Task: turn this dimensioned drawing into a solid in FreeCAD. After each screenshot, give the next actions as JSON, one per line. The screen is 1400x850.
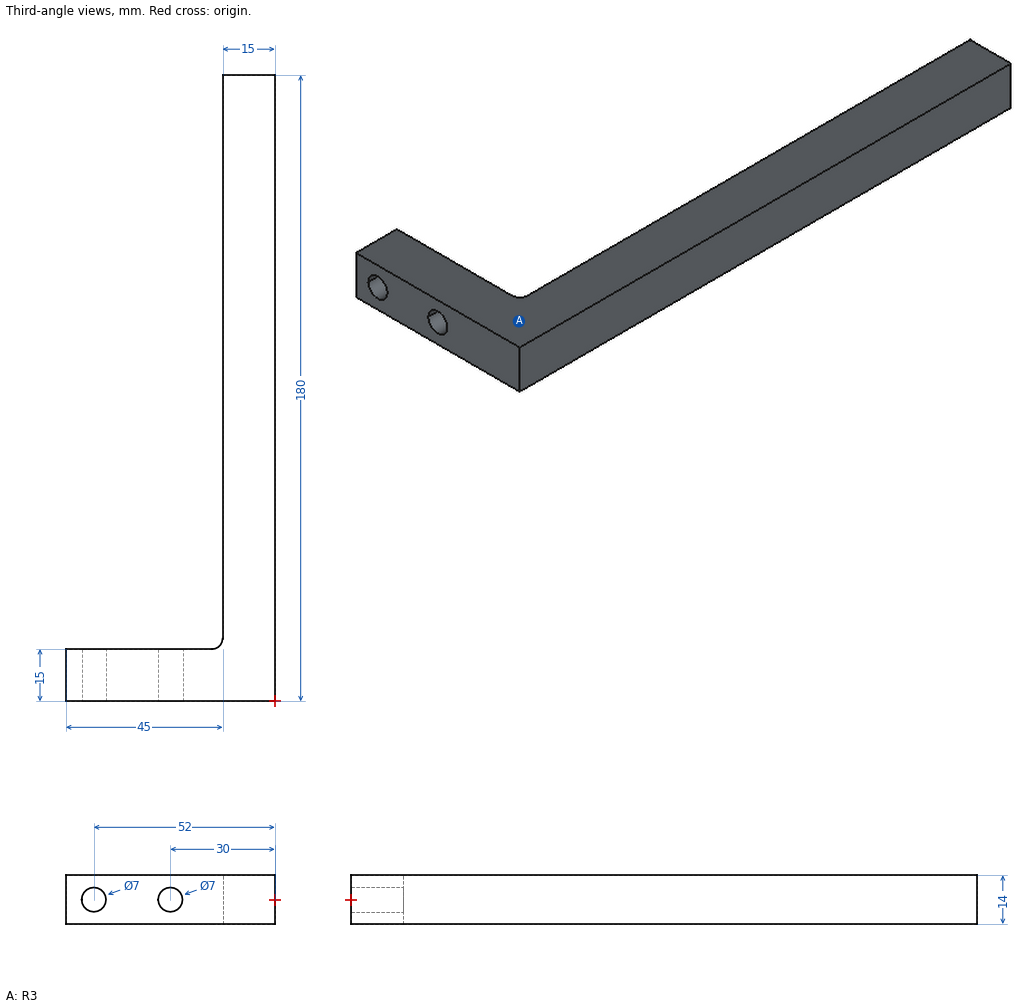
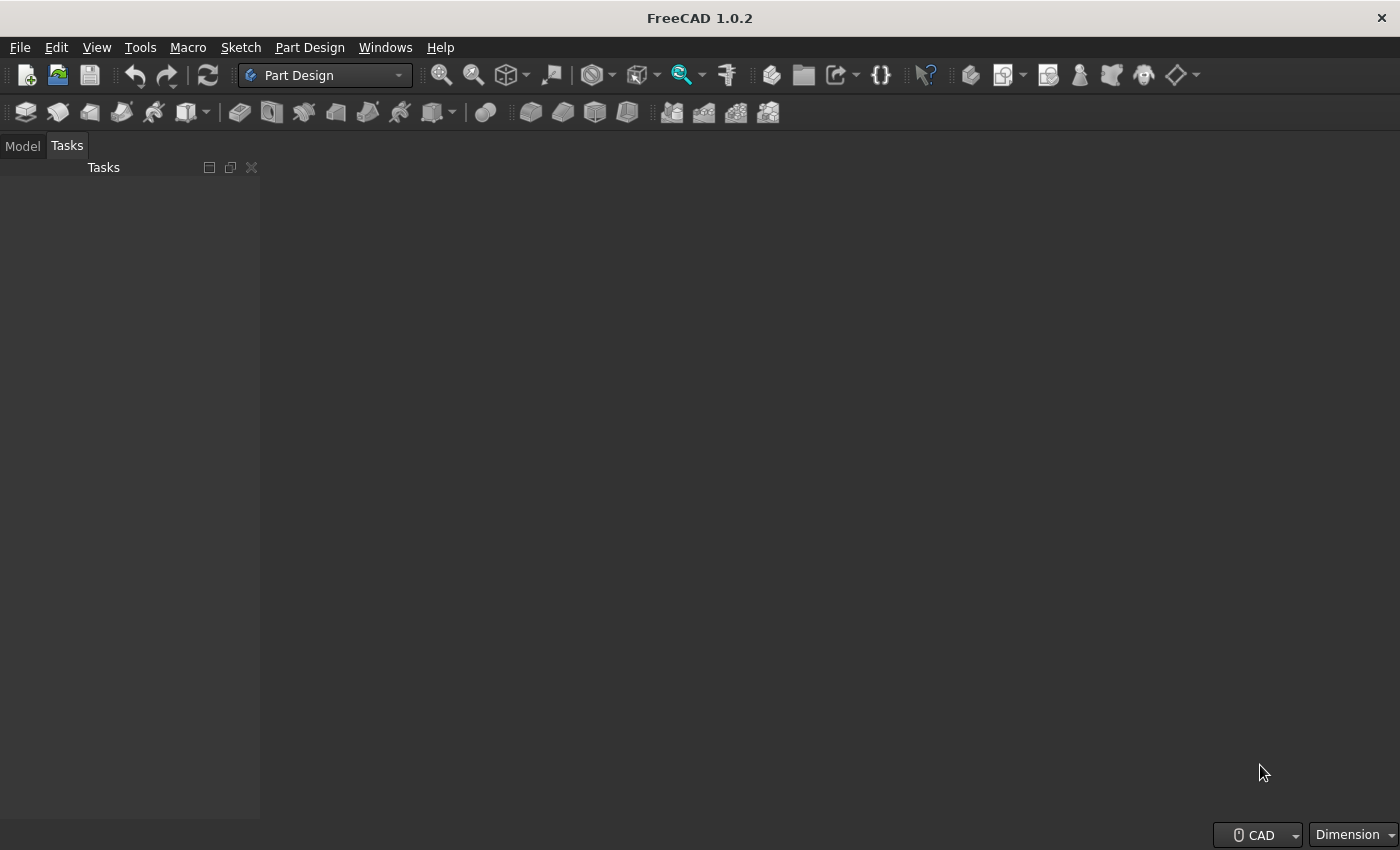
{"action": "left_click", "coordinate": [26, 76]}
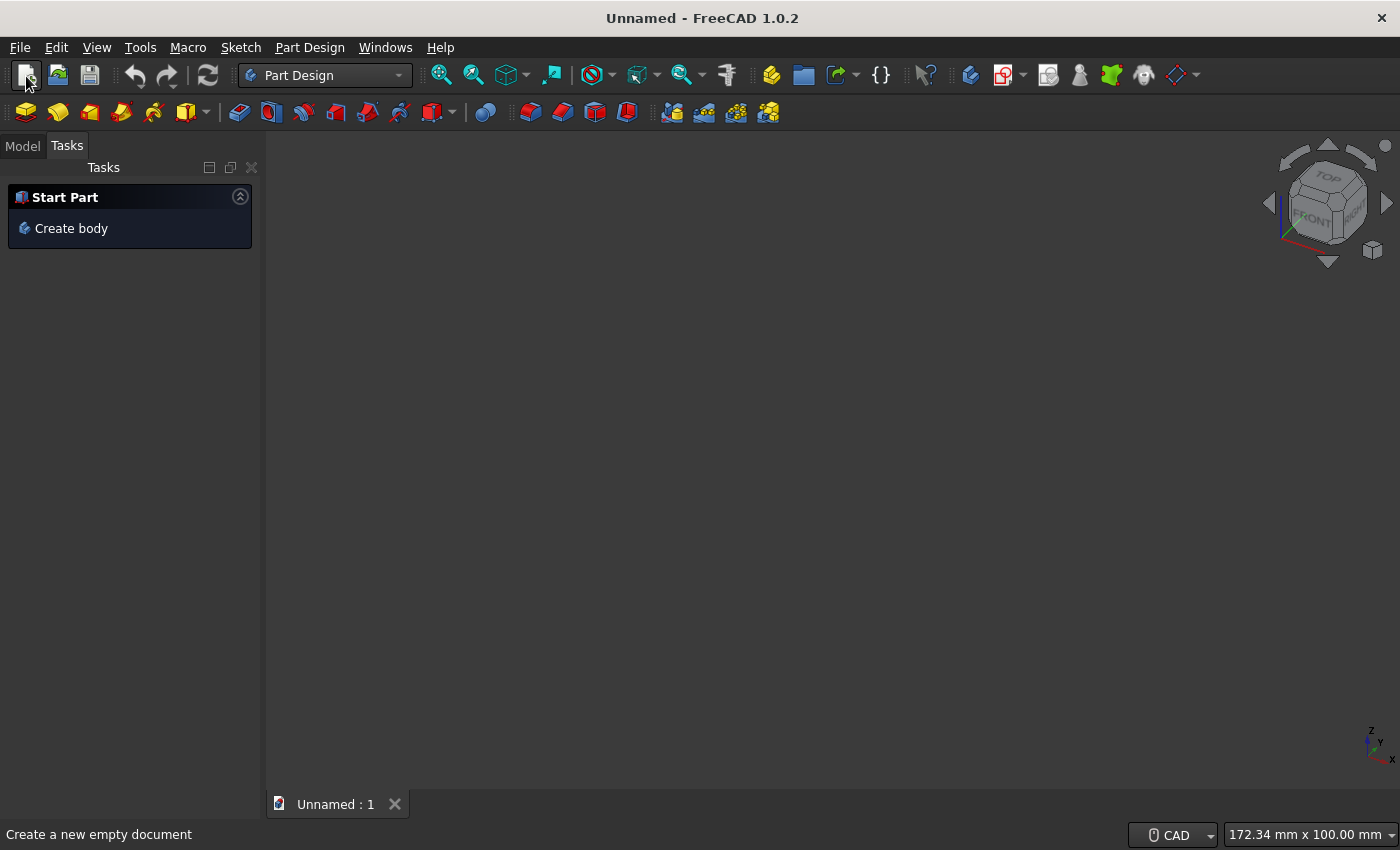
{"action": "left_click", "coordinate": [1004, 76]}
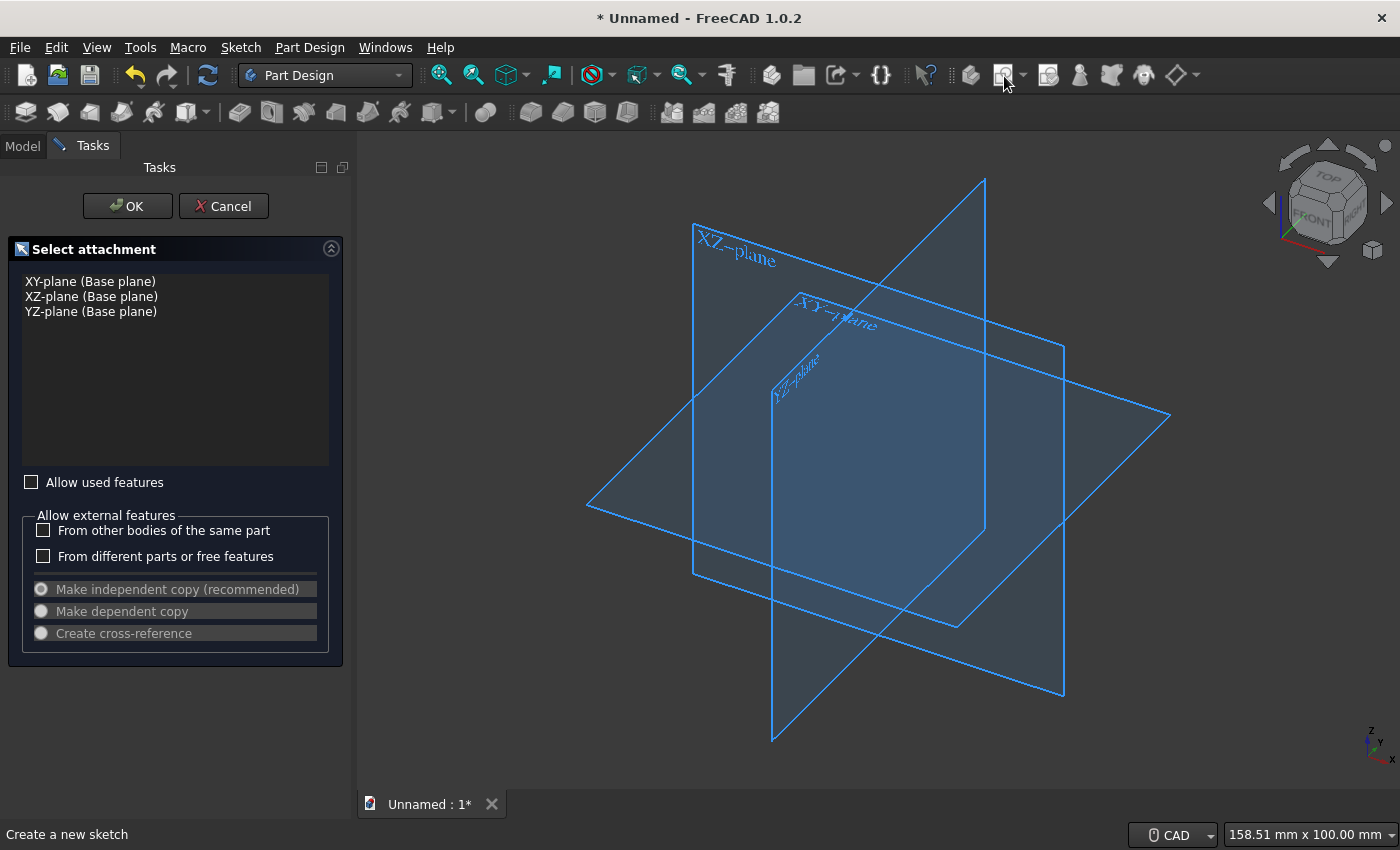
{"action": "left_click", "coordinate": [82, 282]}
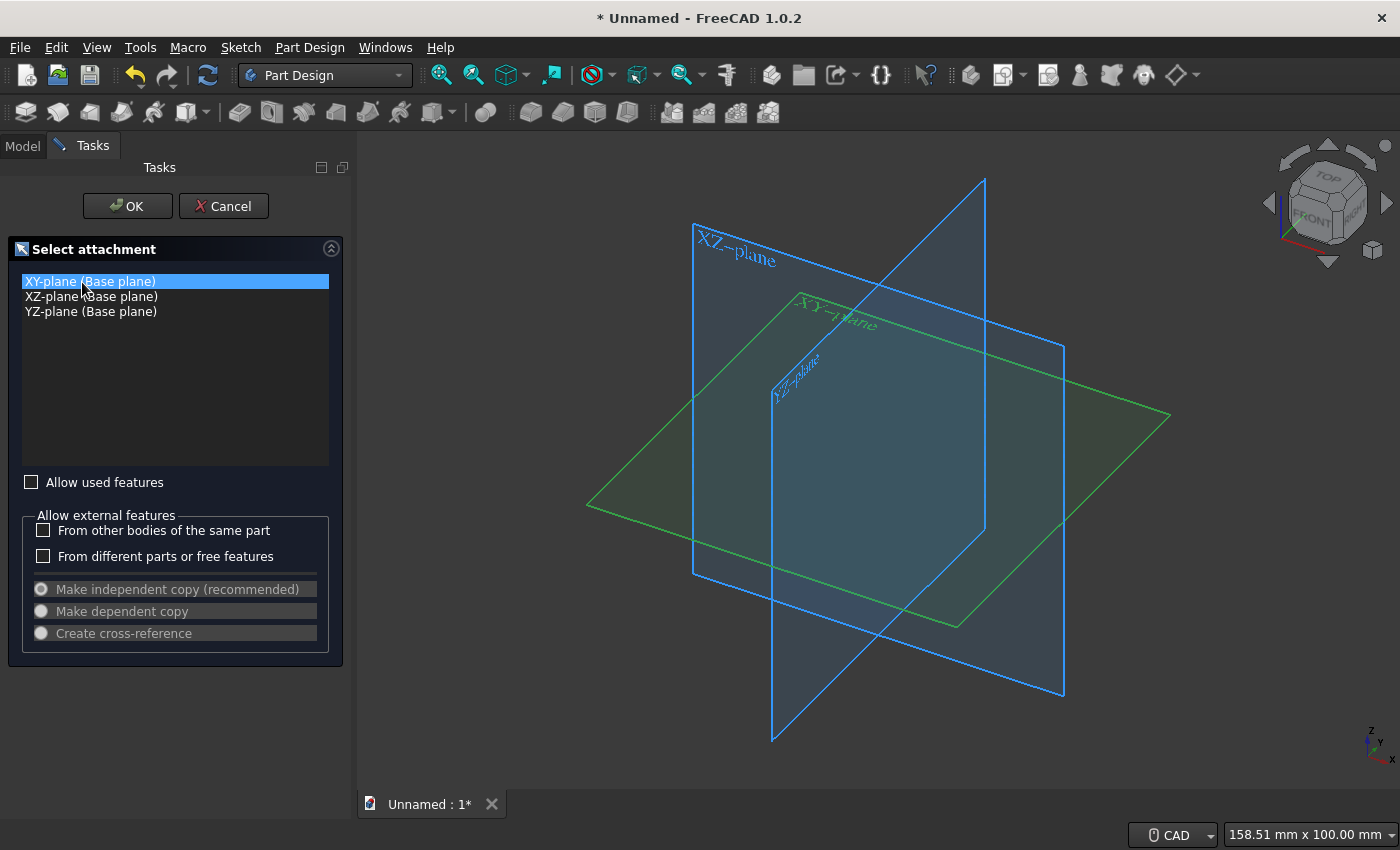
{"action": "left_click", "coordinate": [128, 206]}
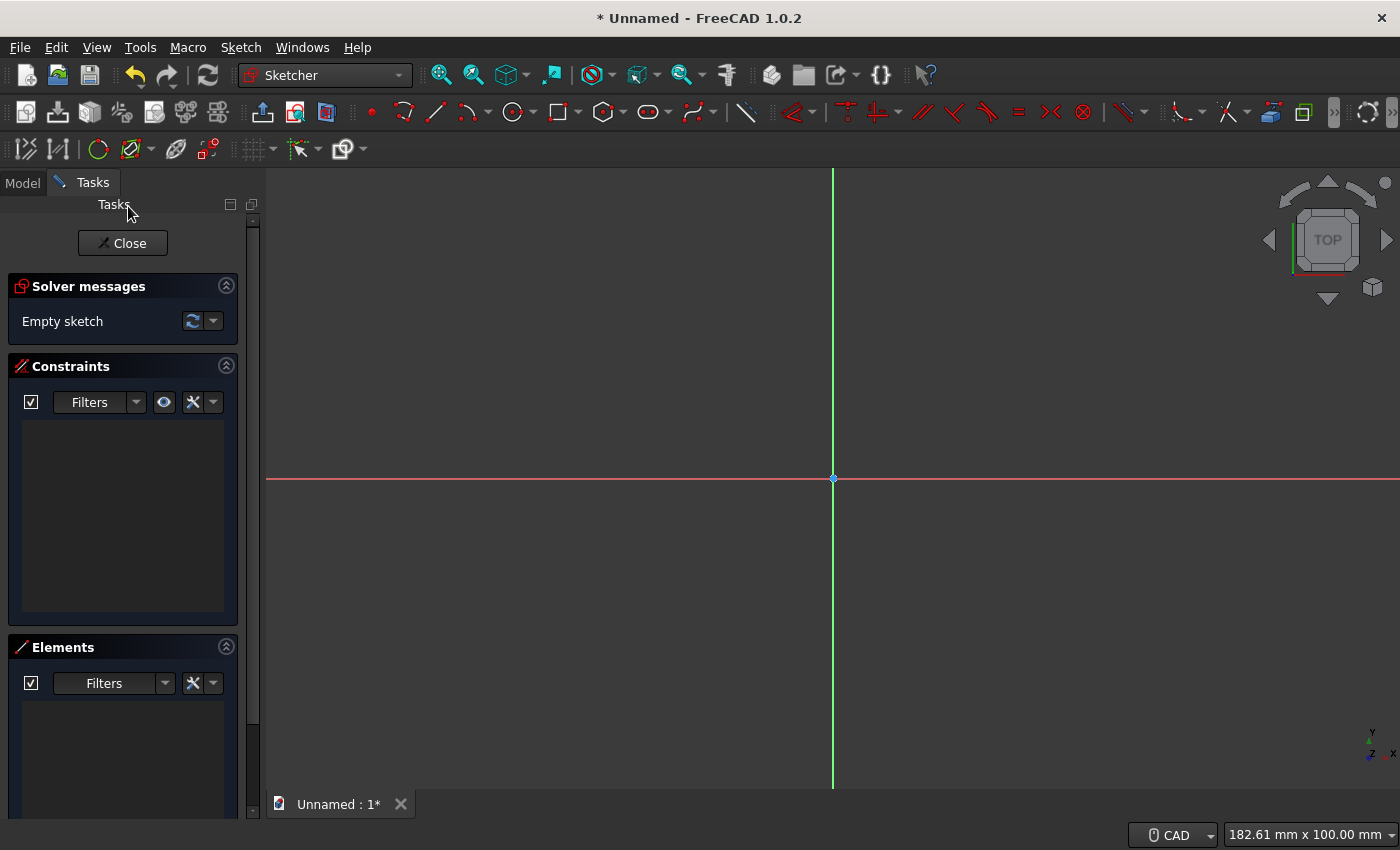
{"action": "scroll", "coordinate": [833, 761], "scroll_direction": "down", "scroll_amount": 5}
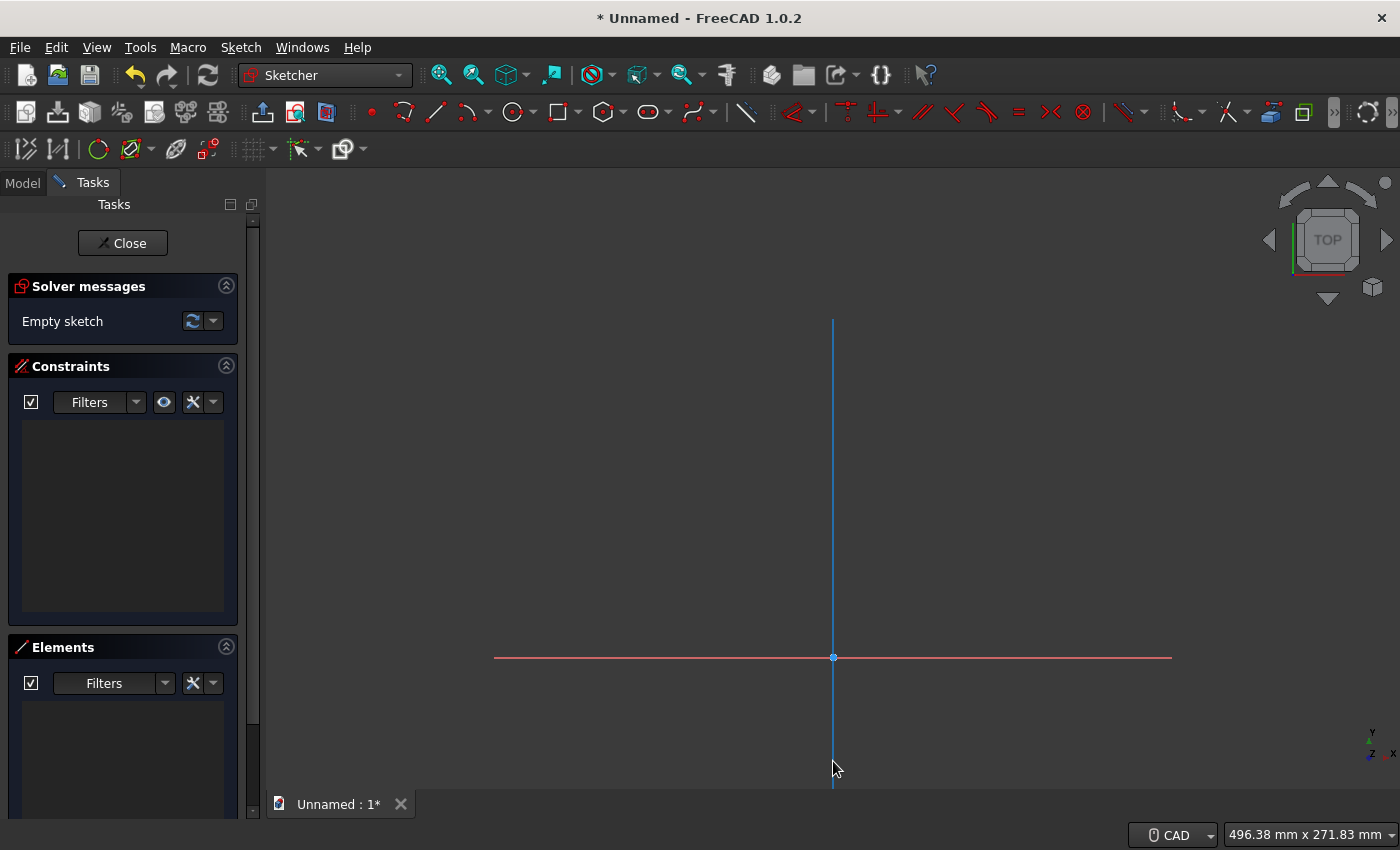
{"action": "left_click", "coordinate": [404, 112]}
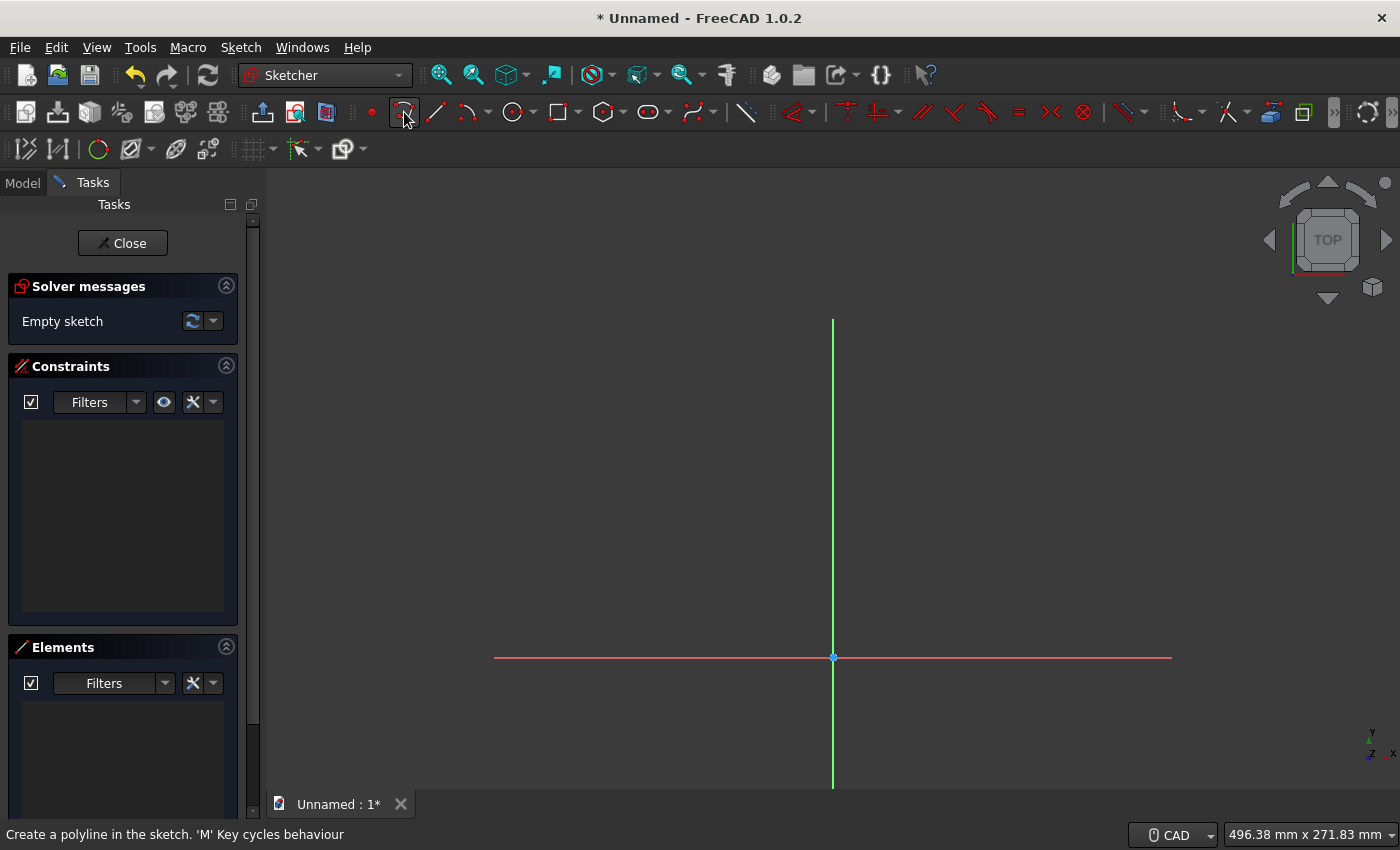
{"action": "left_click", "coordinate": [833, 658]}
{"action": "left_click", "coordinate": [824, 246]}
{"action": "left_click", "coordinate": [799, 246]}
{"action": "left_click", "coordinate": [799, 623]}
{"action": "left_click", "coordinate": [696, 623]}
{"action": "left_click", "coordinate": [696, 649]}
{"action": "left_click", "coordinate": [833, 658]}
{"action": "key", "text": "Escape"}
{"action": "key", "text": "Escape"}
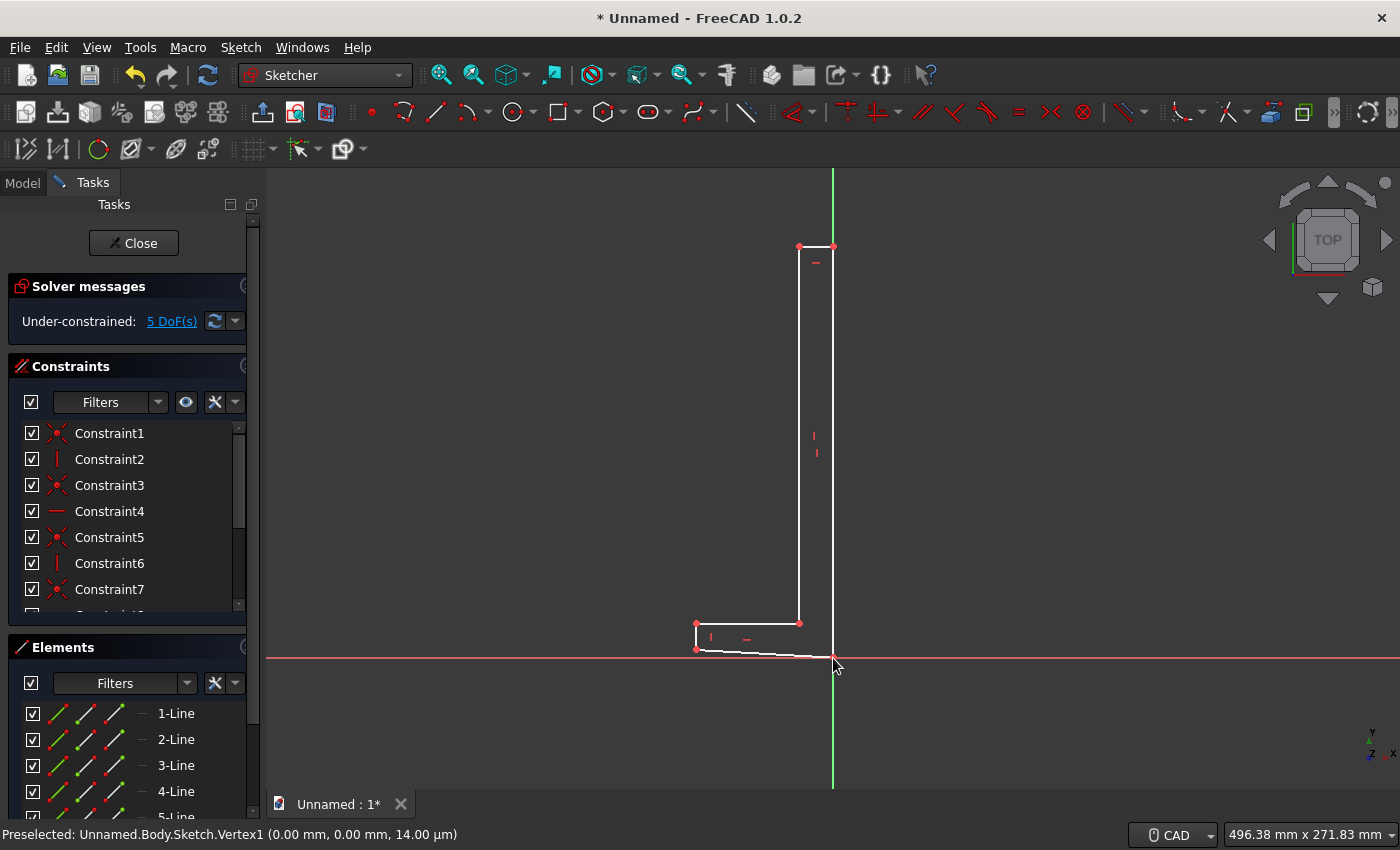
{"action": "left_click", "coordinate": [792, 655]}